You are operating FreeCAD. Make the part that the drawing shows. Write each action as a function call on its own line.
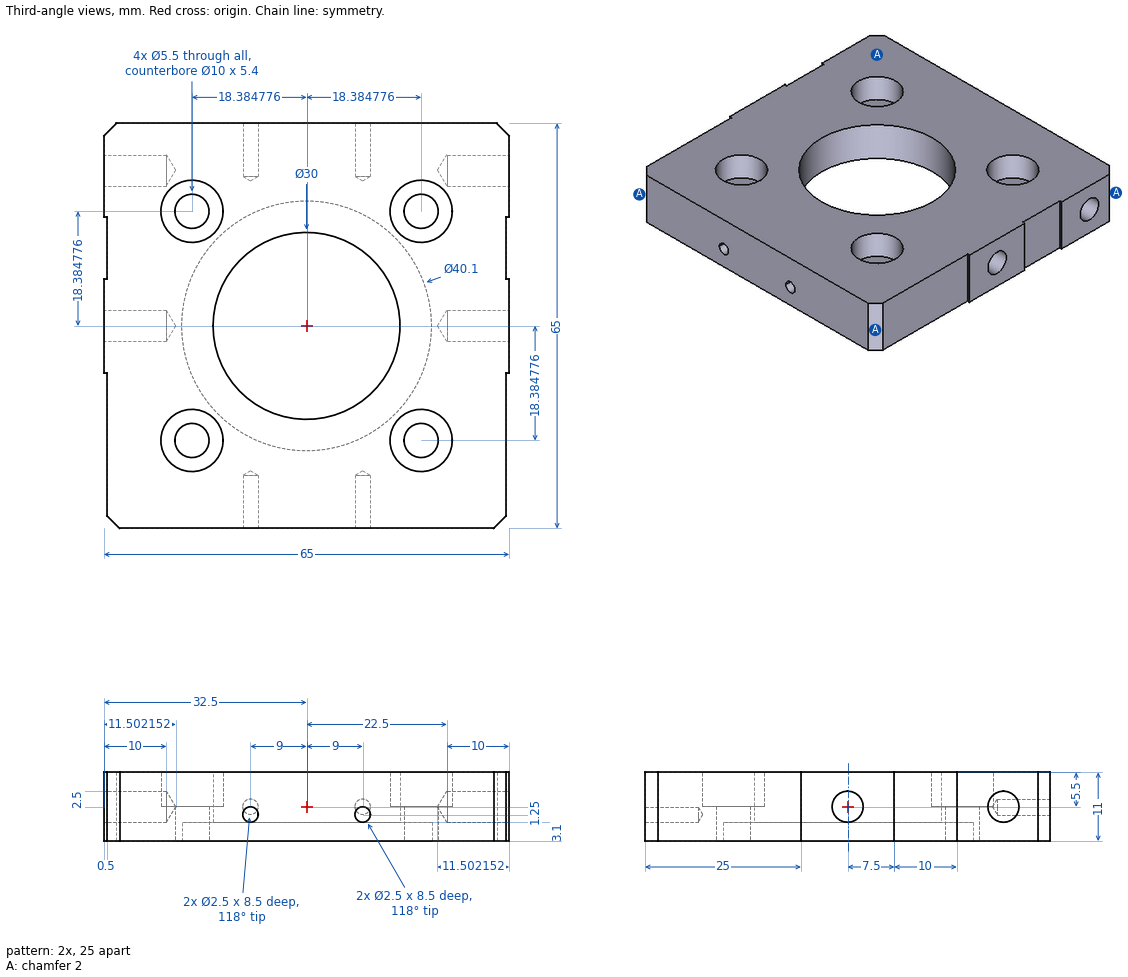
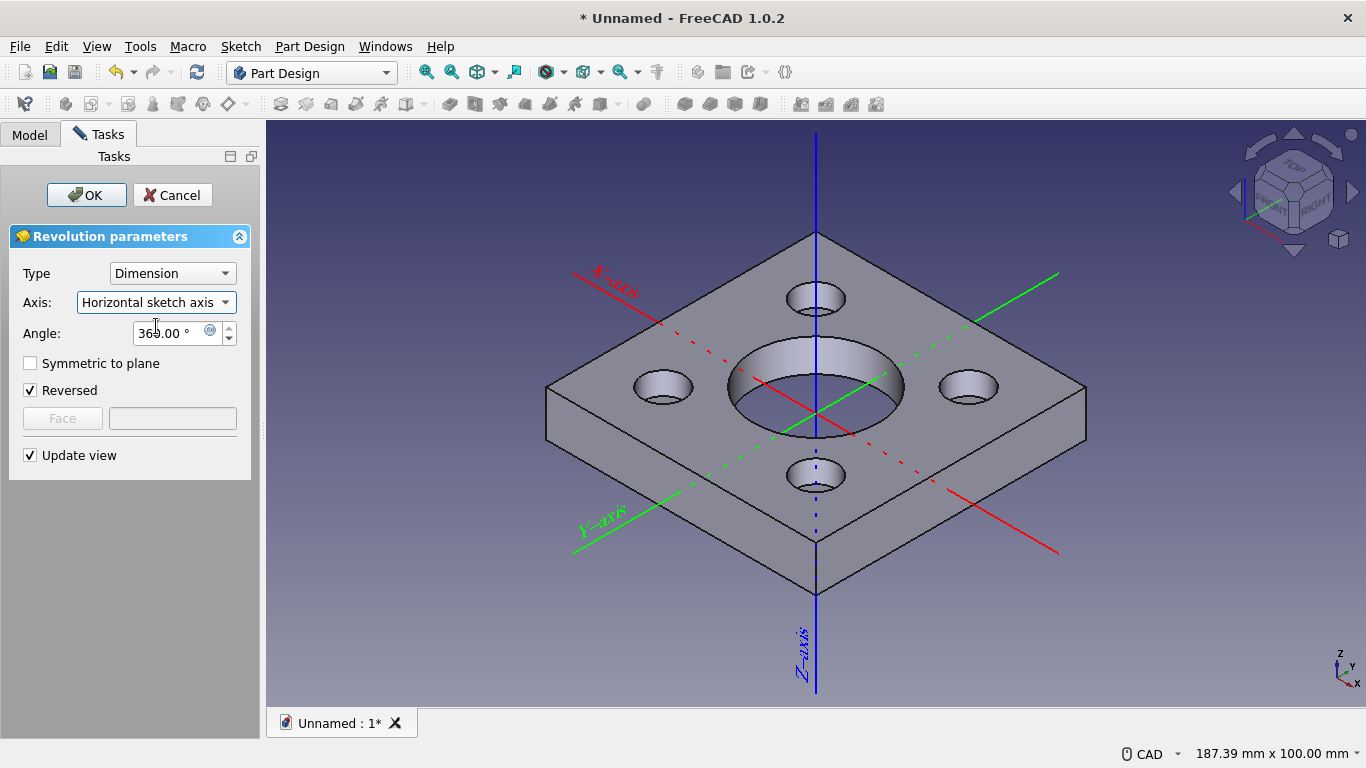
click(87, 195)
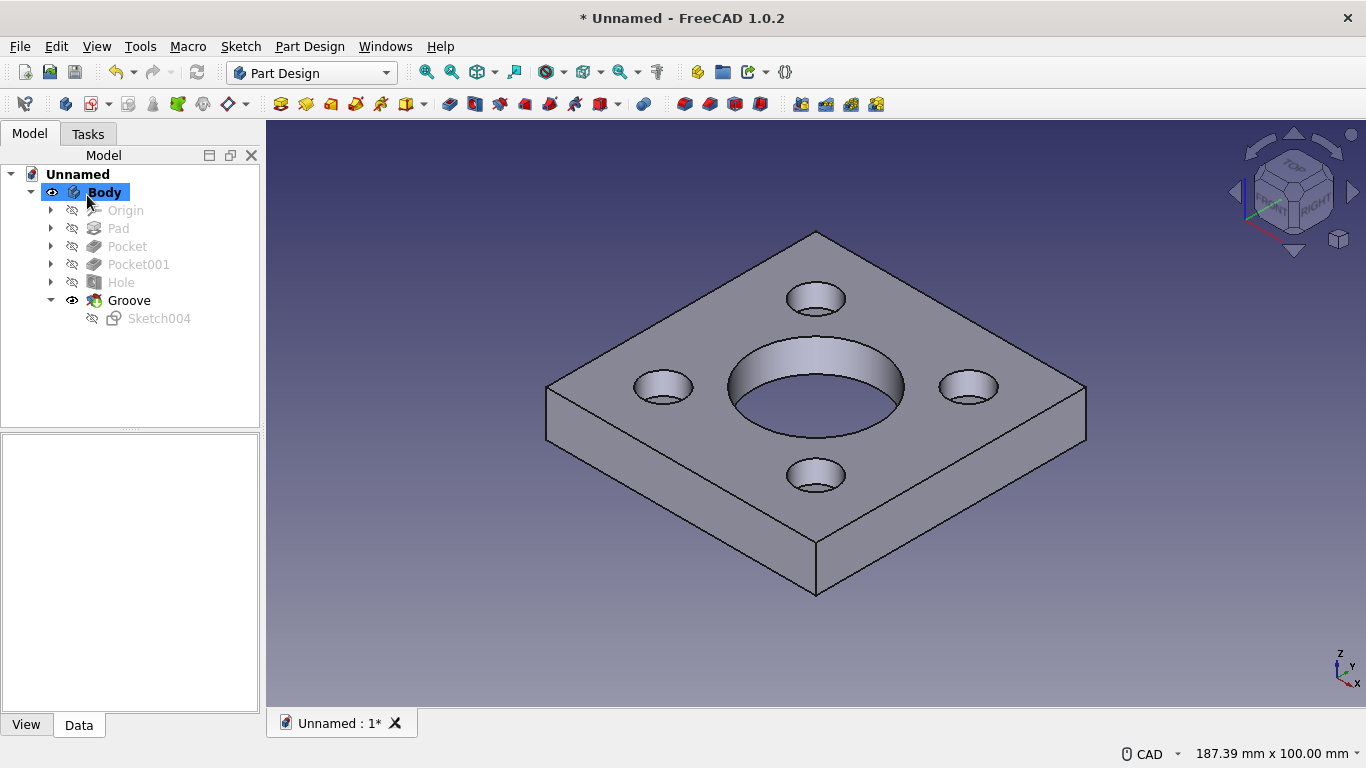
click(117, 300)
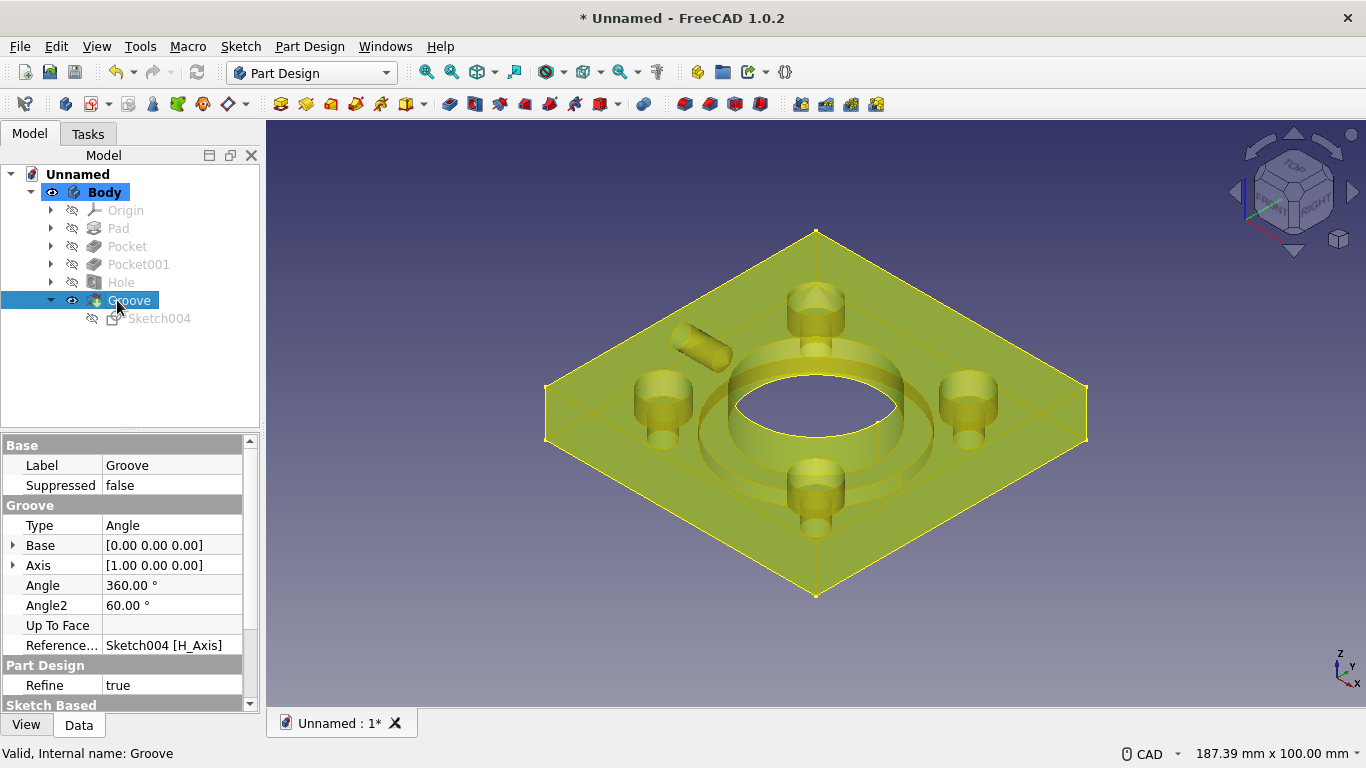
click(826, 104)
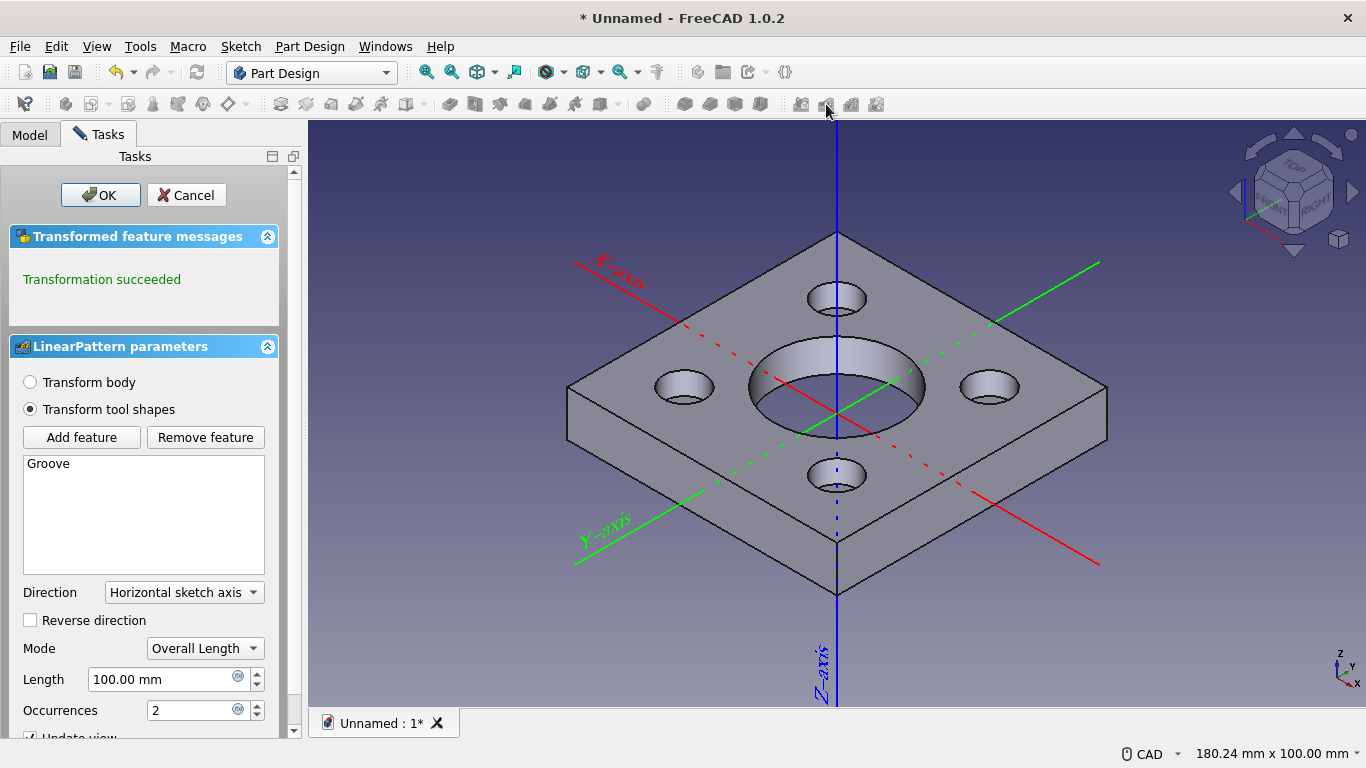
click(185, 592)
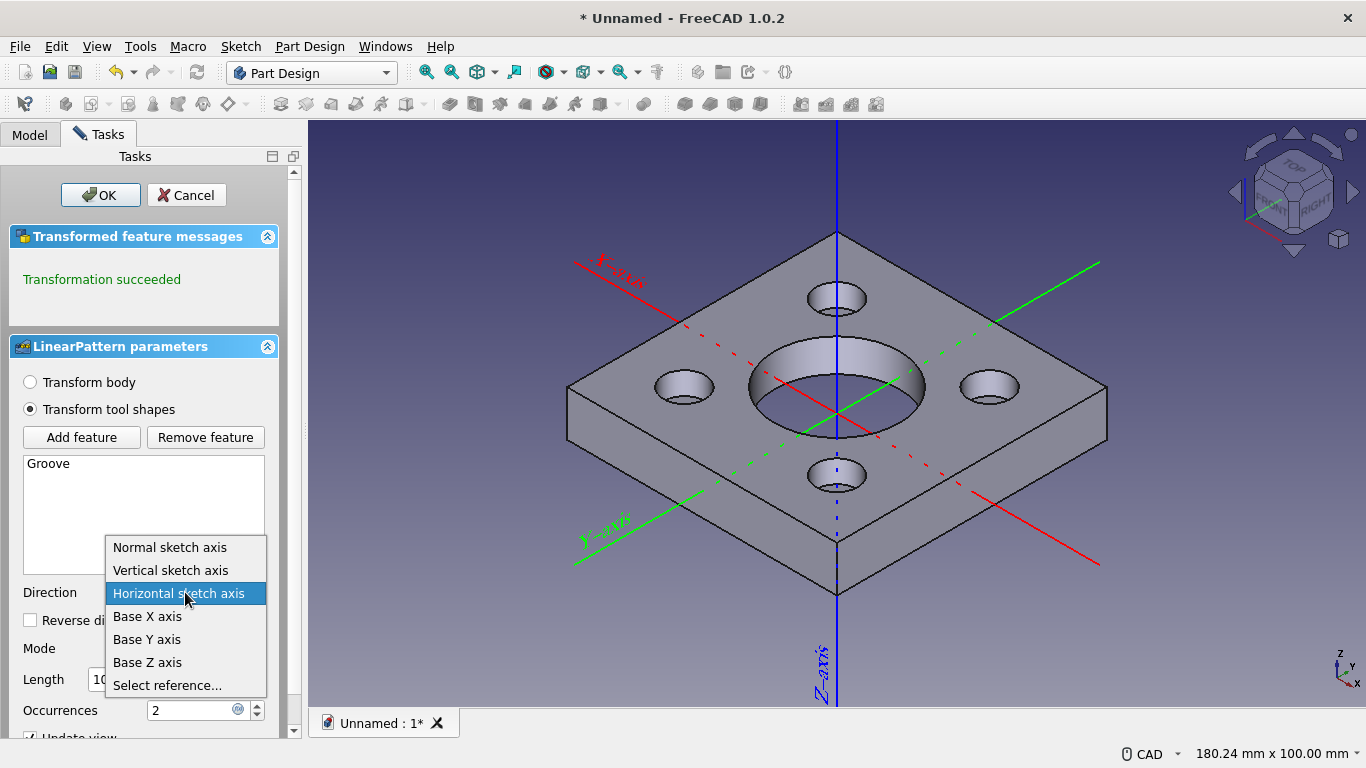
click(184, 640)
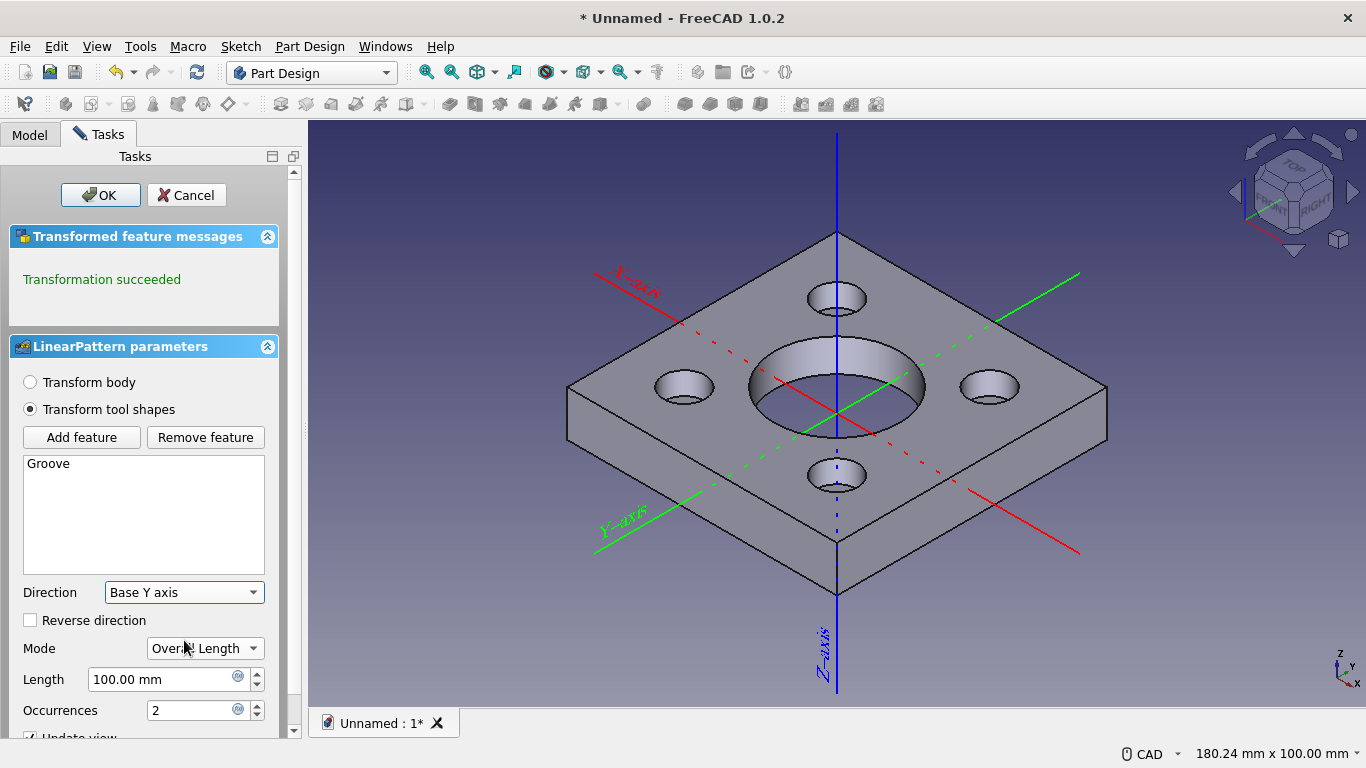
click(206, 648)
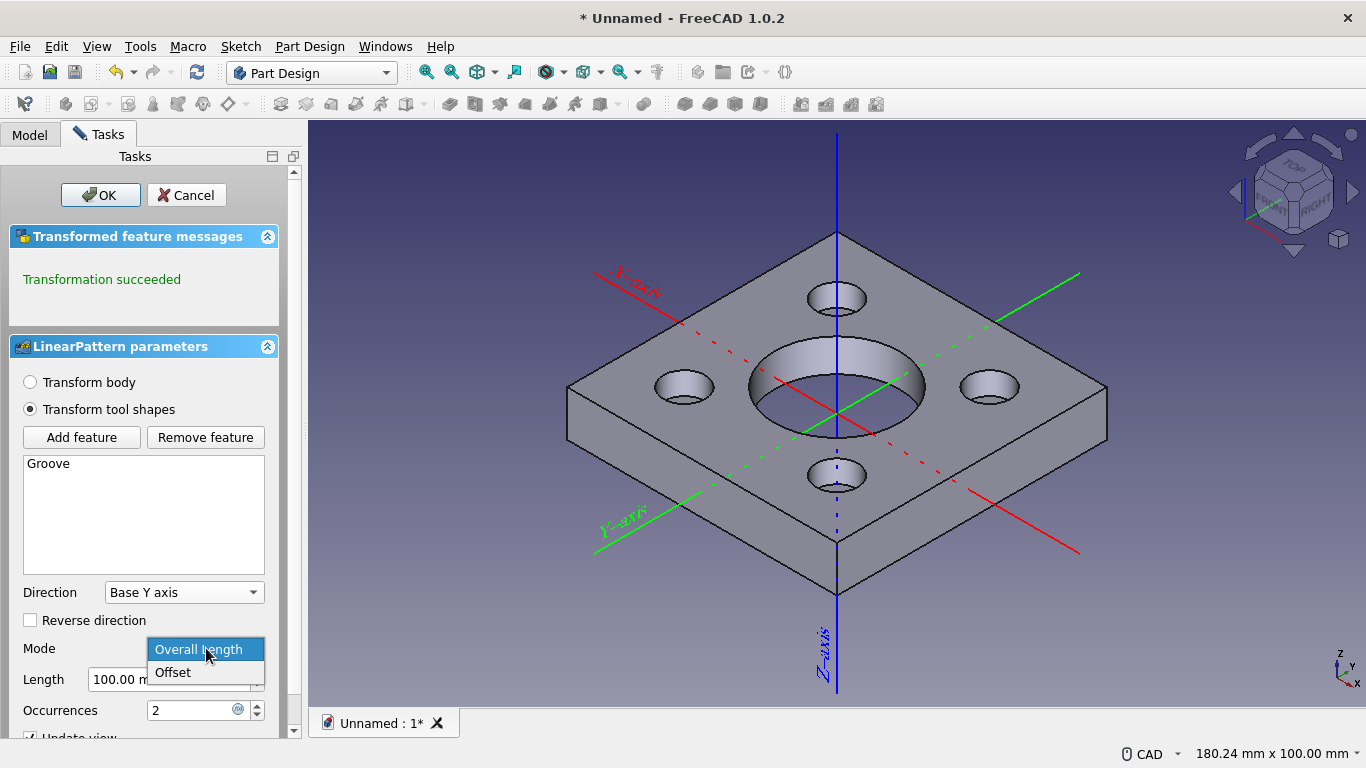
click(204, 672)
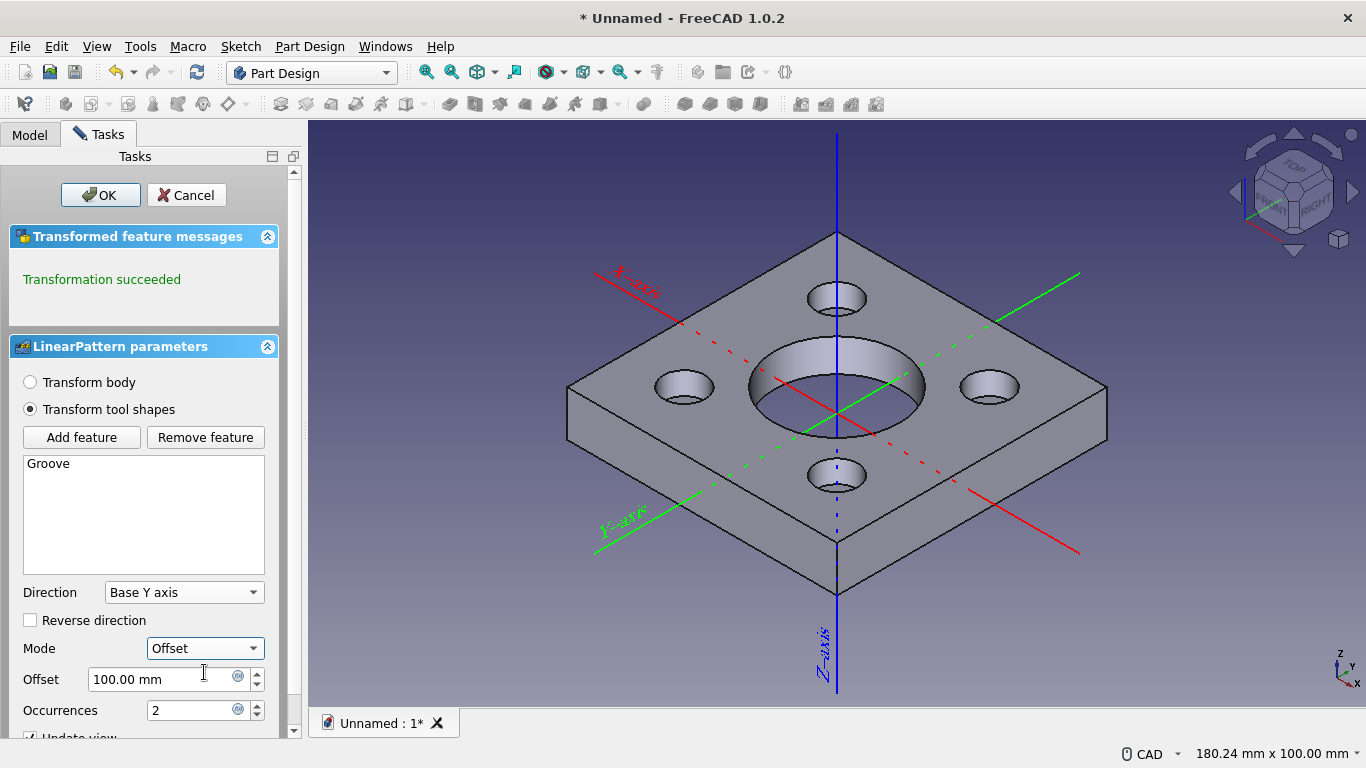
triple_click(170, 680)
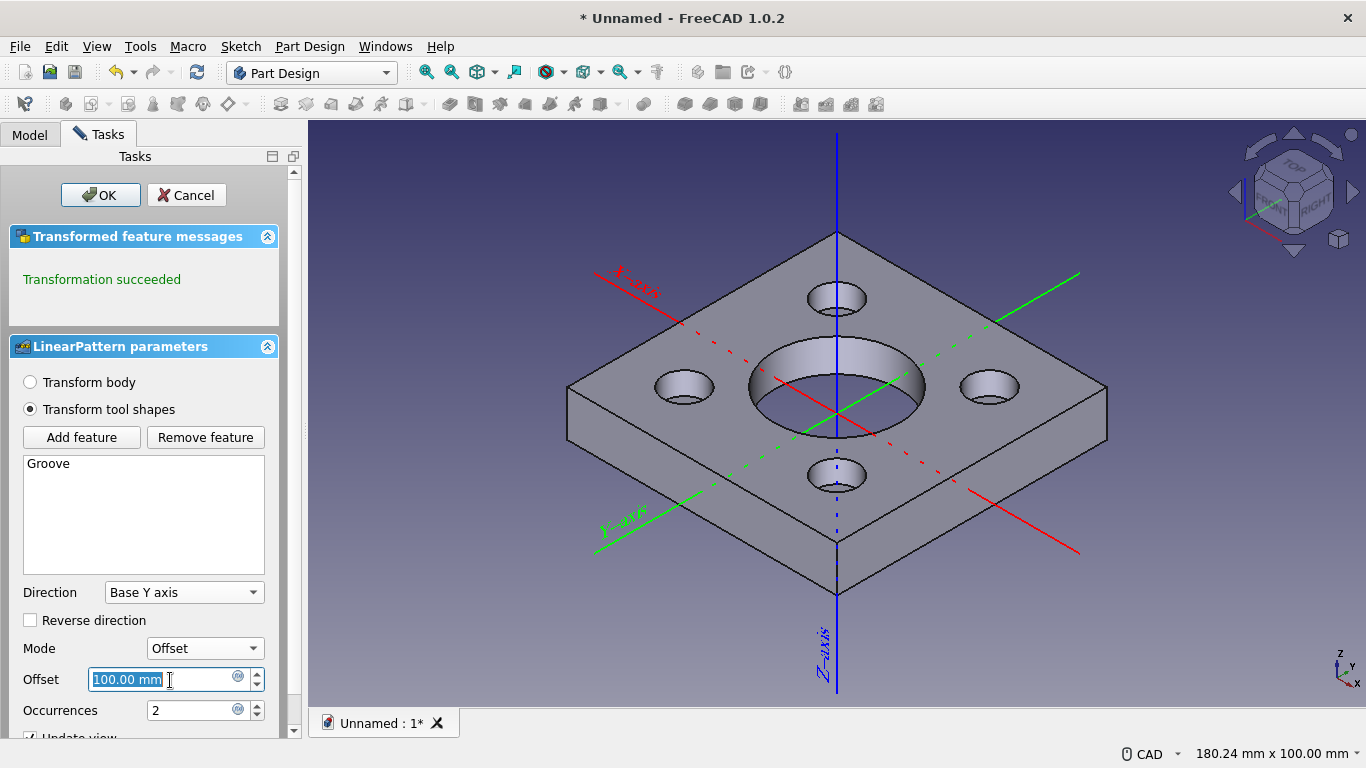
text(25)
key(Tab)